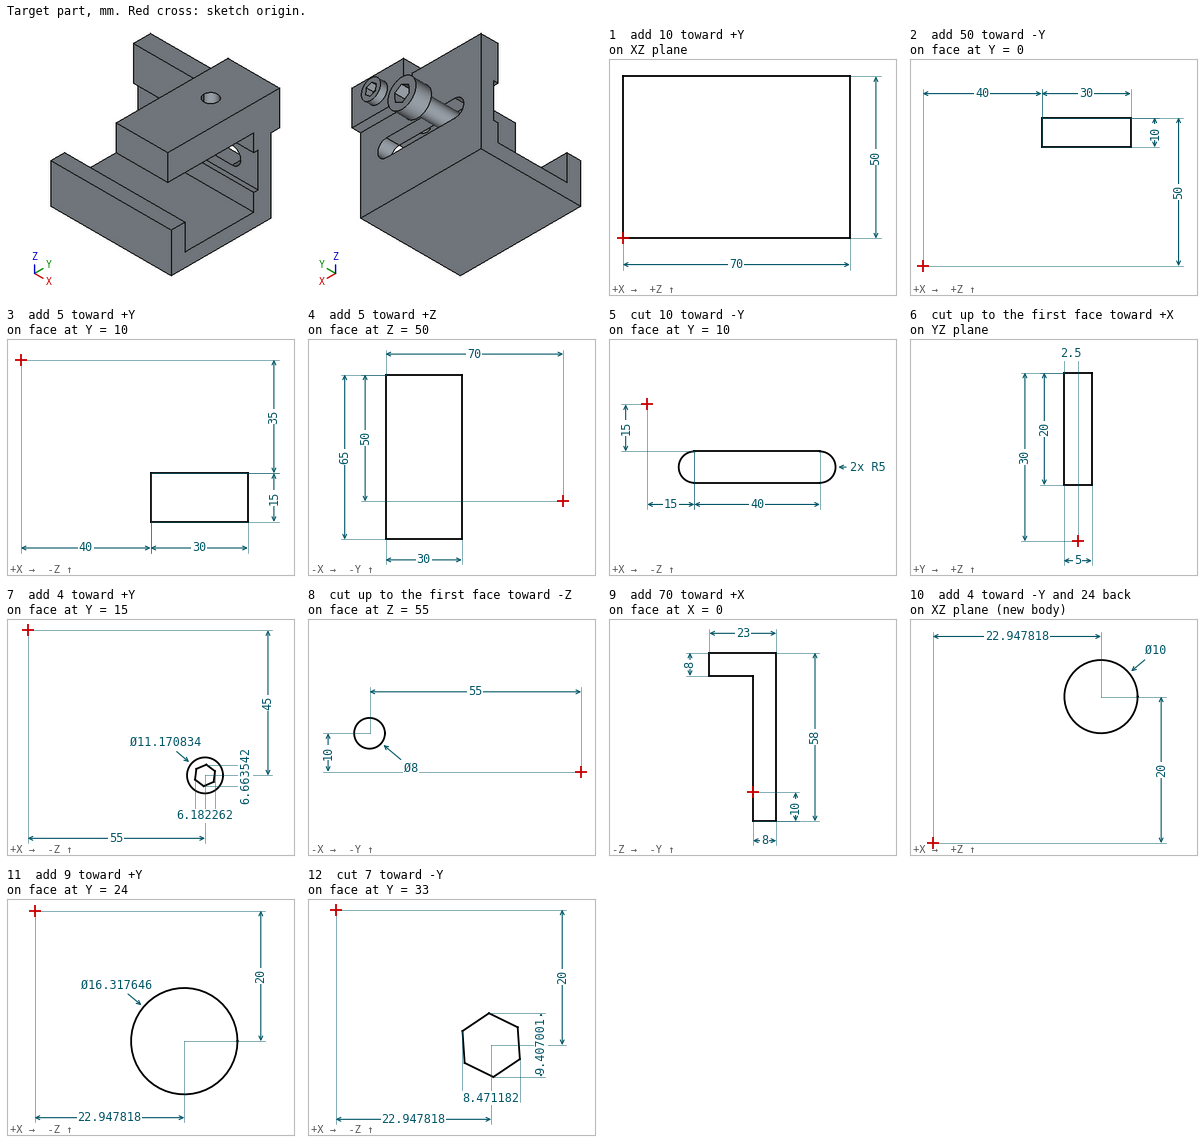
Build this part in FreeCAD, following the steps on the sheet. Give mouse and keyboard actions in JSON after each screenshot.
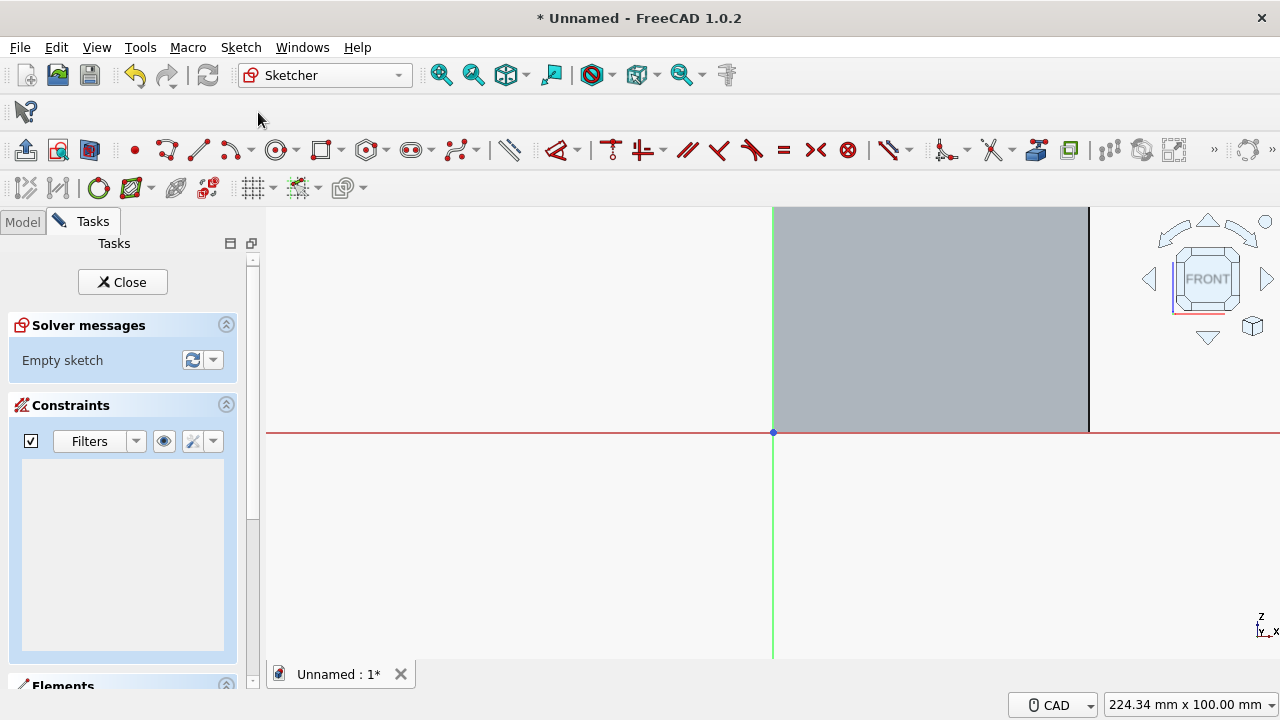
{"action": "scroll", "coordinate": [294, 631], "scroll_direction": "down", "scroll_amount": 1}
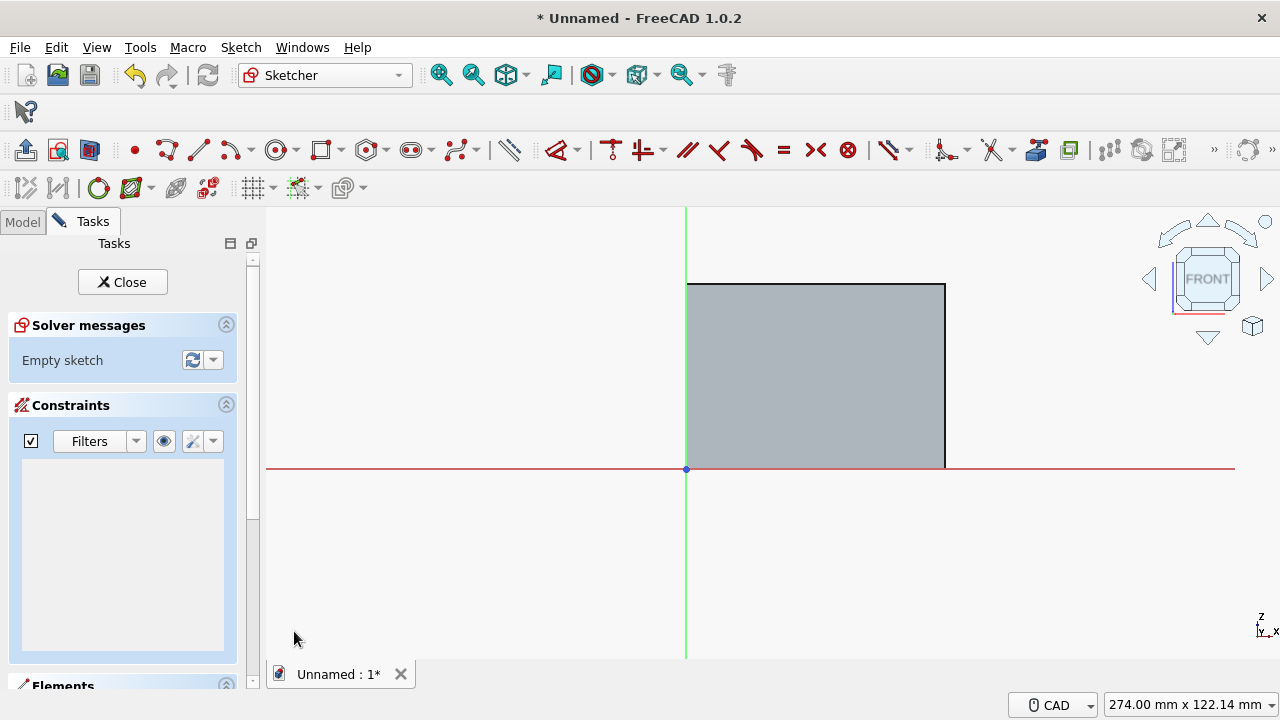
{"action": "scroll", "coordinate": [1042, 262], "scroll_direction": "up", "scroll_amount": 2}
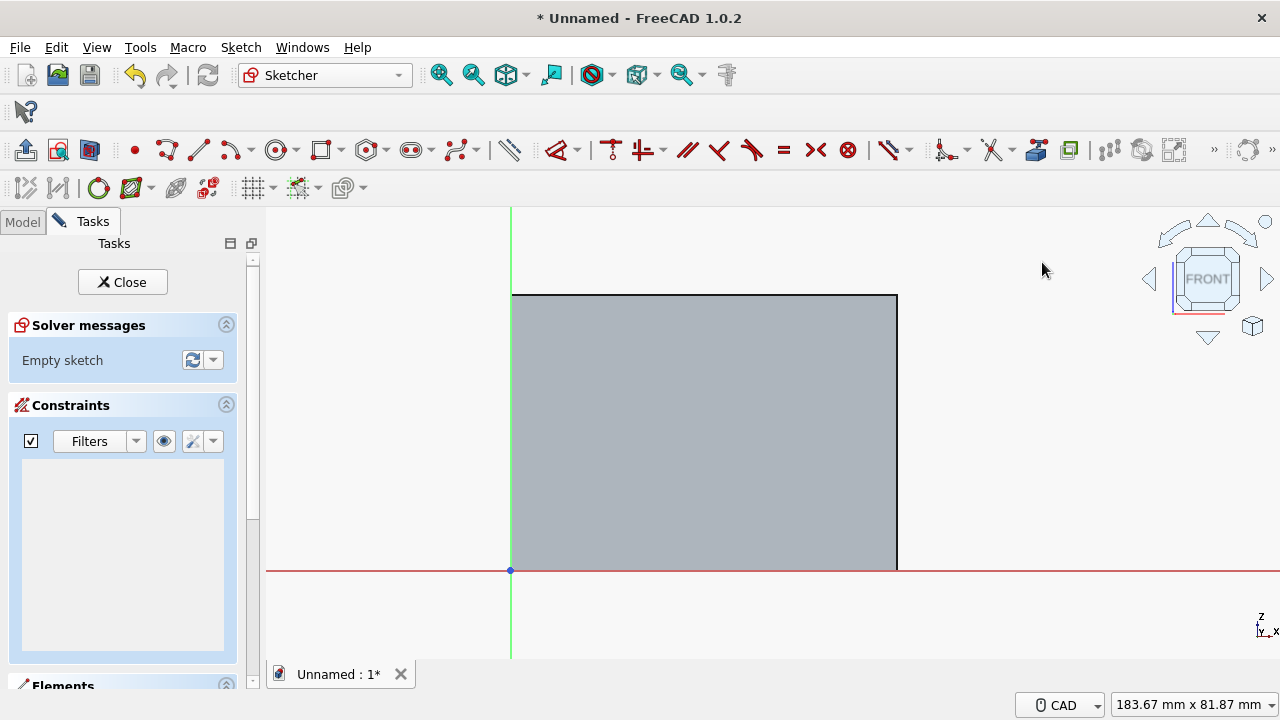
{"action": "left_click", "coordinate": [322, 150]}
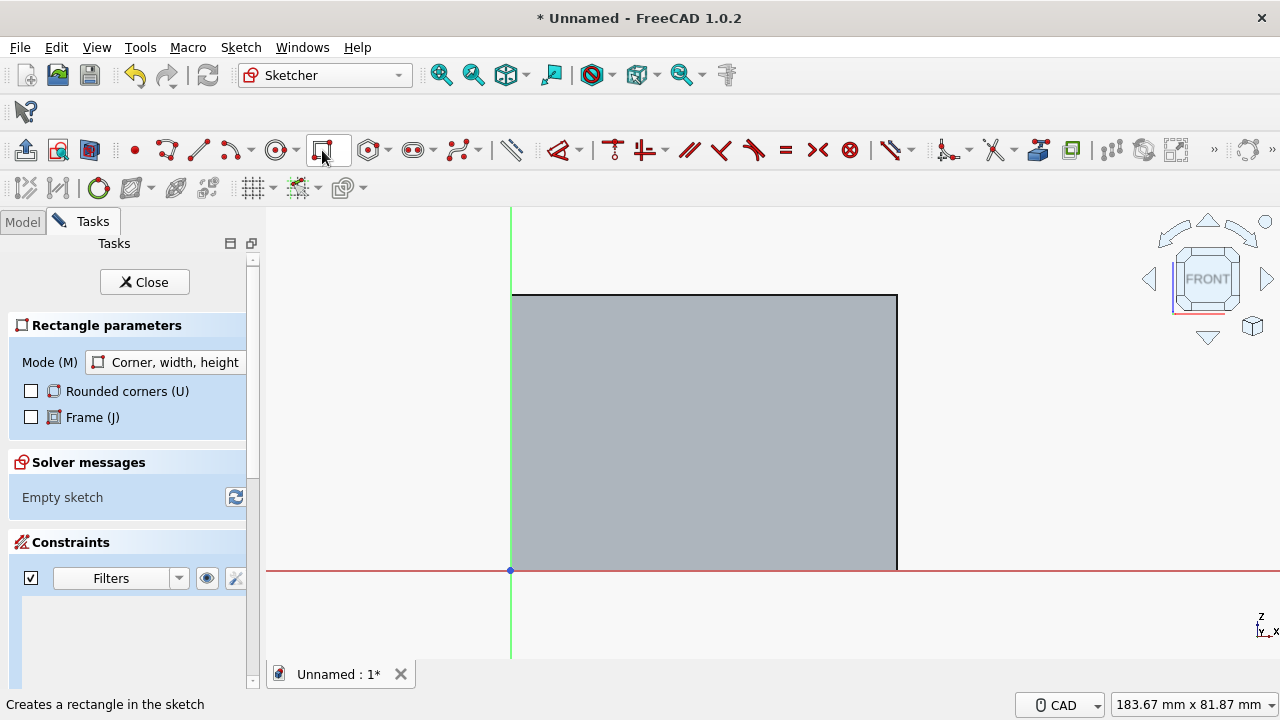
{"action": "left_click", "coordinate": [732, 295]}
{"action": "left_click", "coordinate": [897, 350]}
{"action": "key", "text": "Escape"}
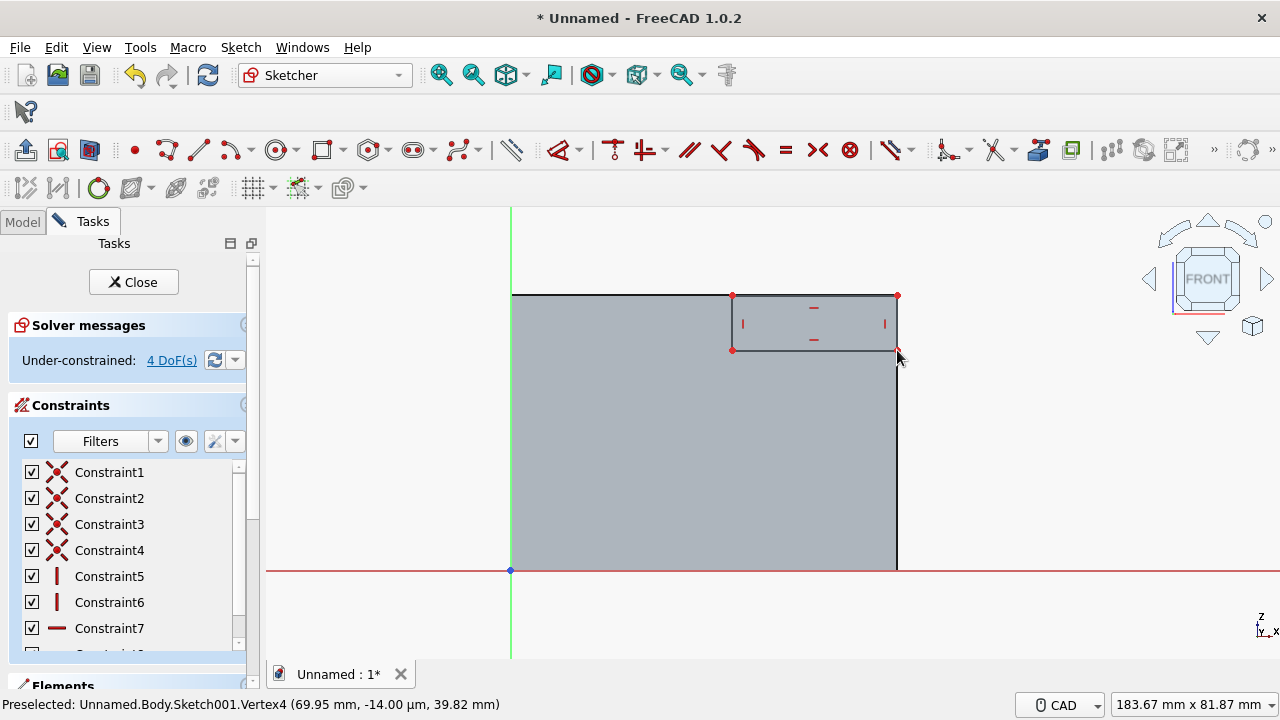
{"action": "left_click", "coordinate": [558, 150]}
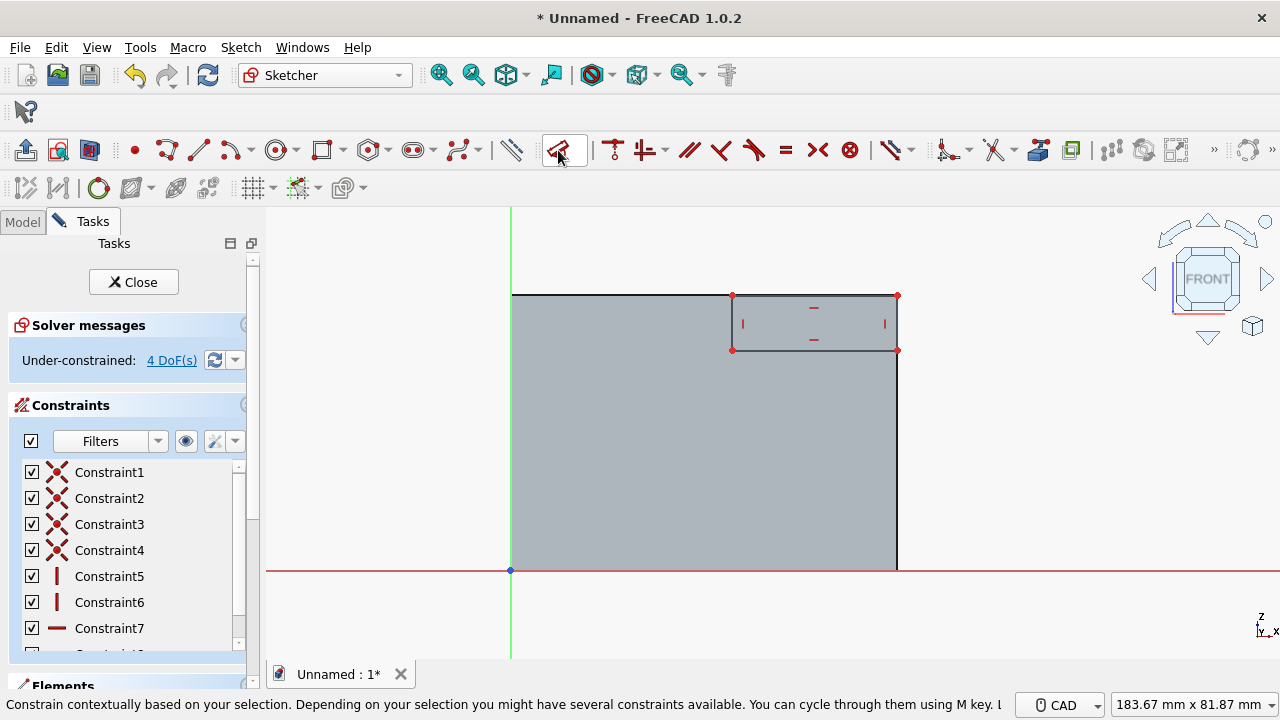
{"action": "left_click", "coordinate": [732, 312]}
{"action": "left_click", "coordinate": [766, 323]}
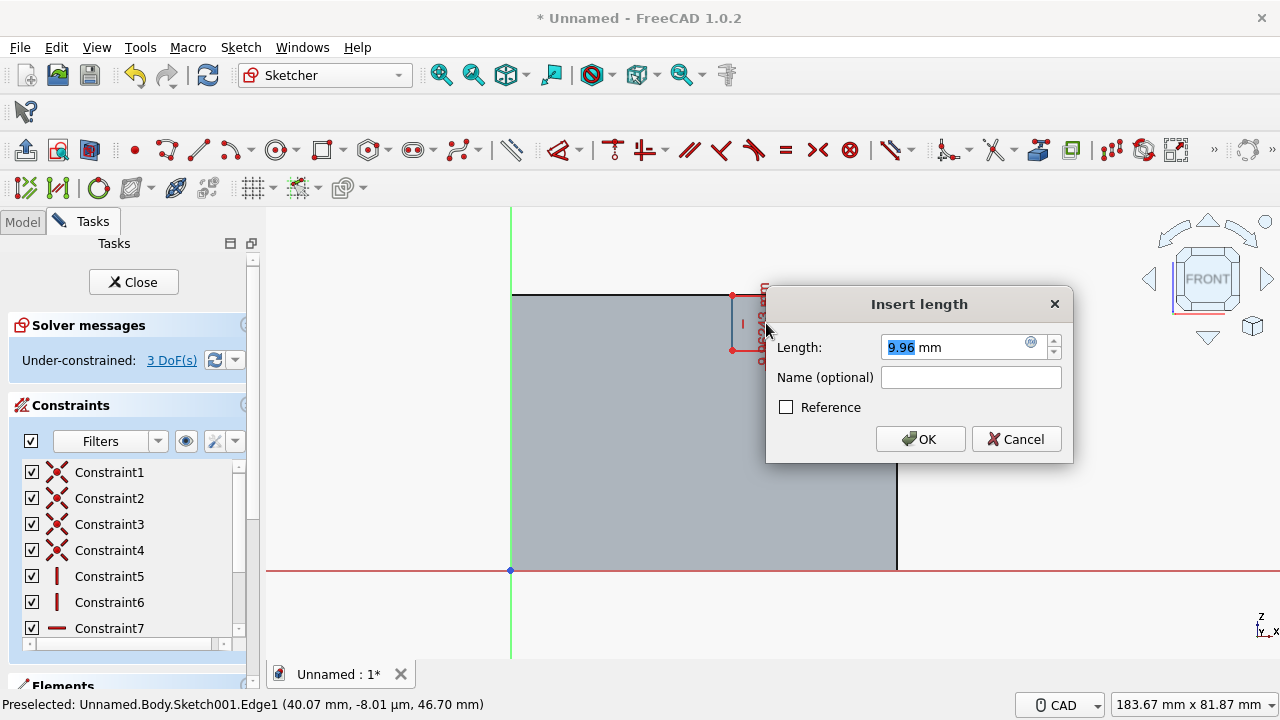
{"action": "type", "text": "10"}
{"action": "key", "text": "Return"}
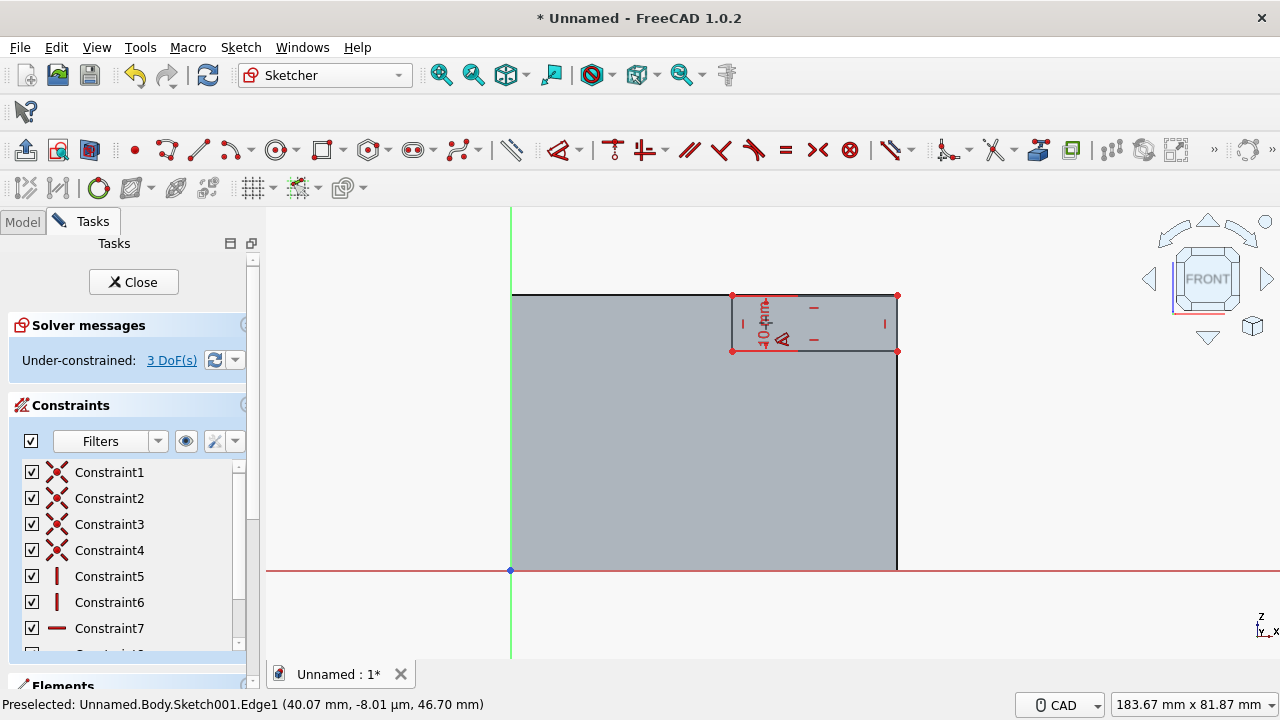
{"action": "left_click", "coordinate": [782, 351]}
{"action": "left_click", "coordinate": [852, 317]}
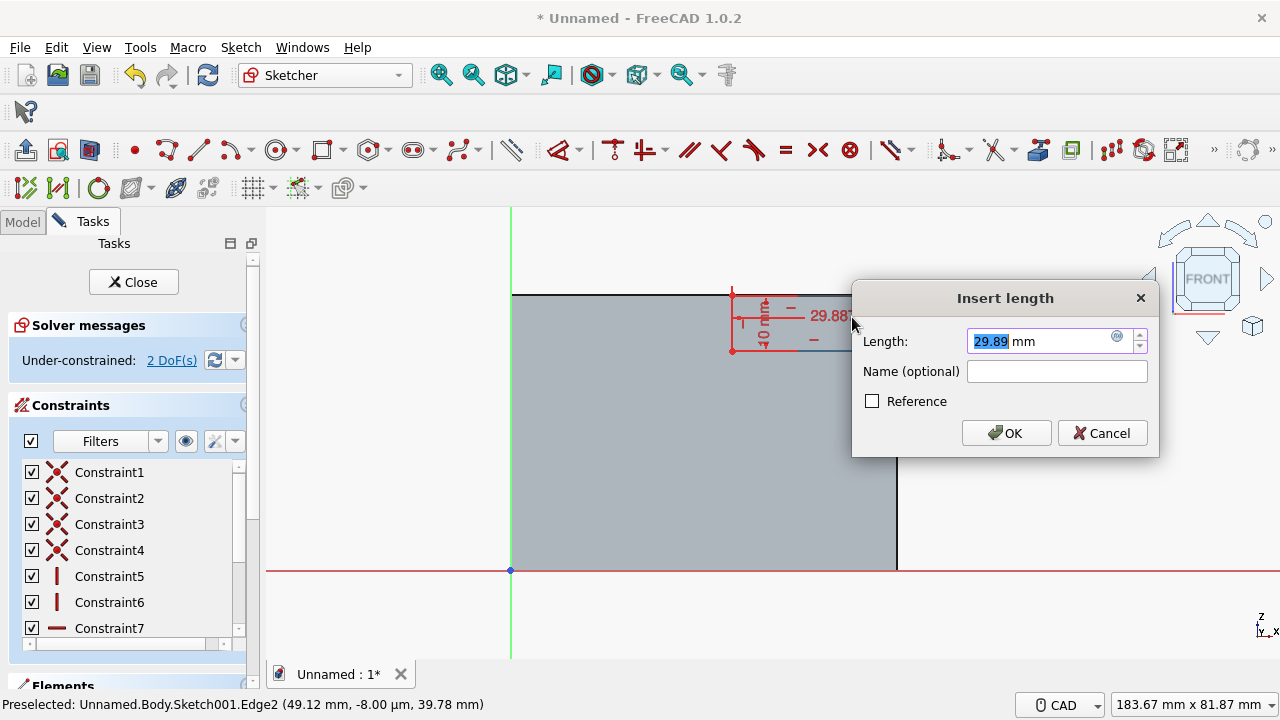
{"action": "type", "text": "30"}
{"action": "key", "text": "Return"}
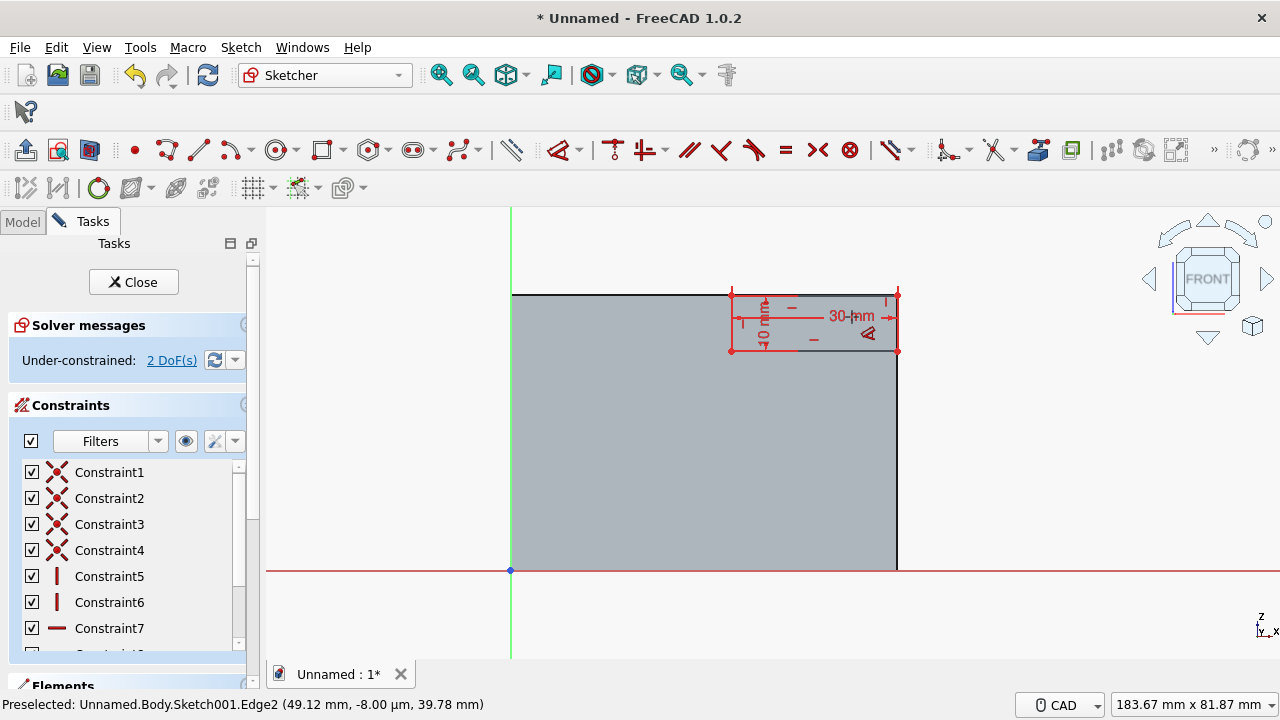
{"action": "left_click", "coordinate": [732, 296]}
{"action": "left_click", "coordinate": [621, 605]}